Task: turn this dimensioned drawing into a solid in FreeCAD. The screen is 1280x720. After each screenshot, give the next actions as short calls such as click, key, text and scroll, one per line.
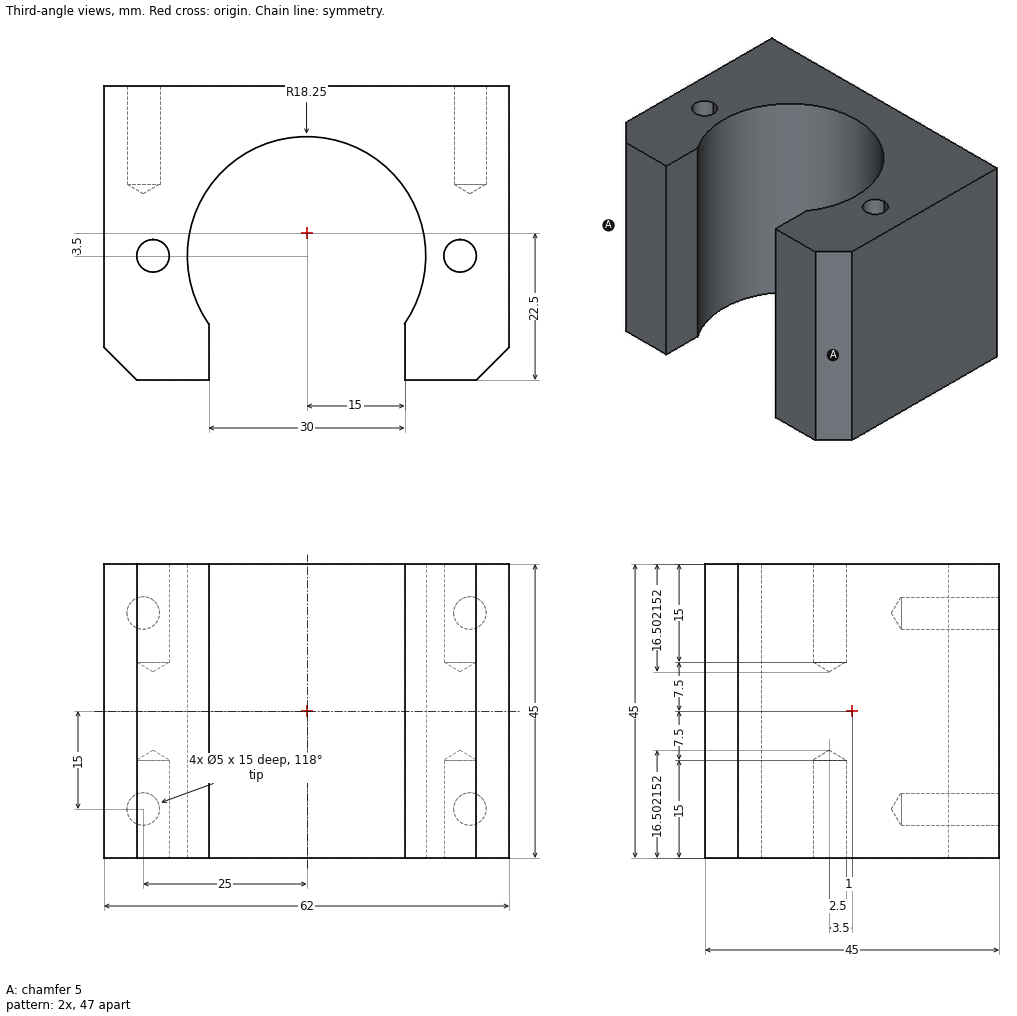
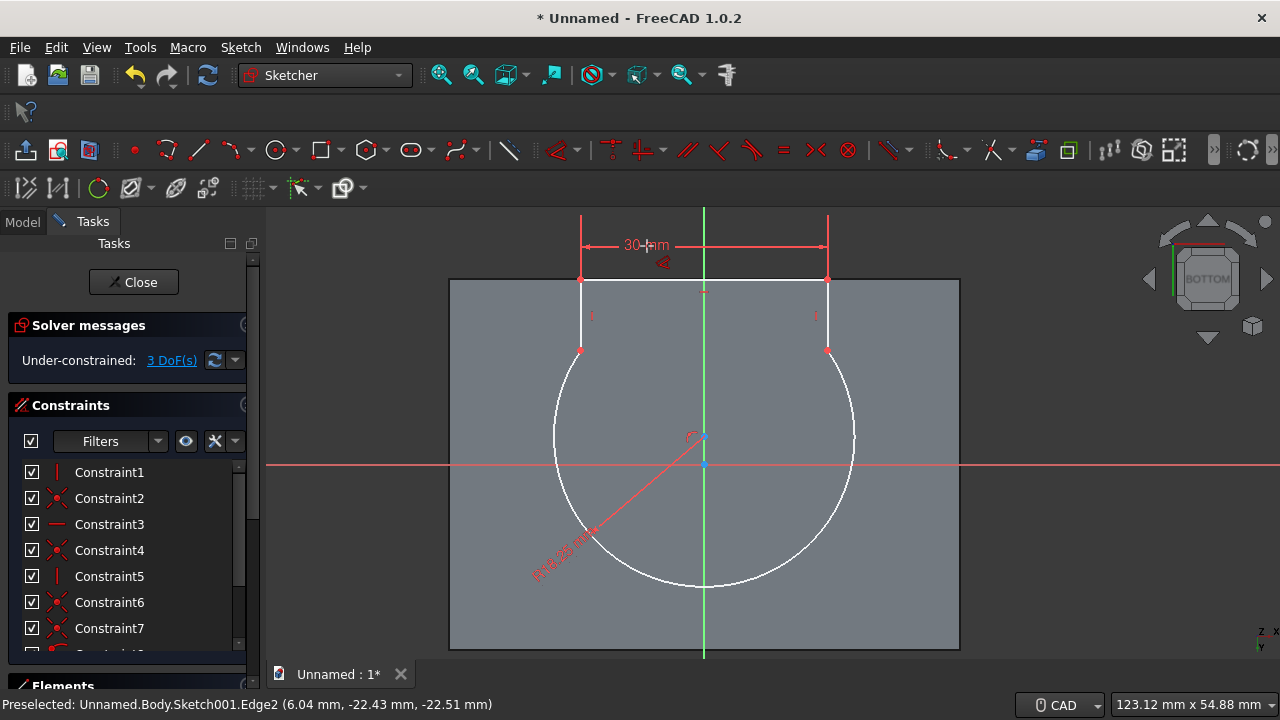
click(828, 351)
click(766, 317)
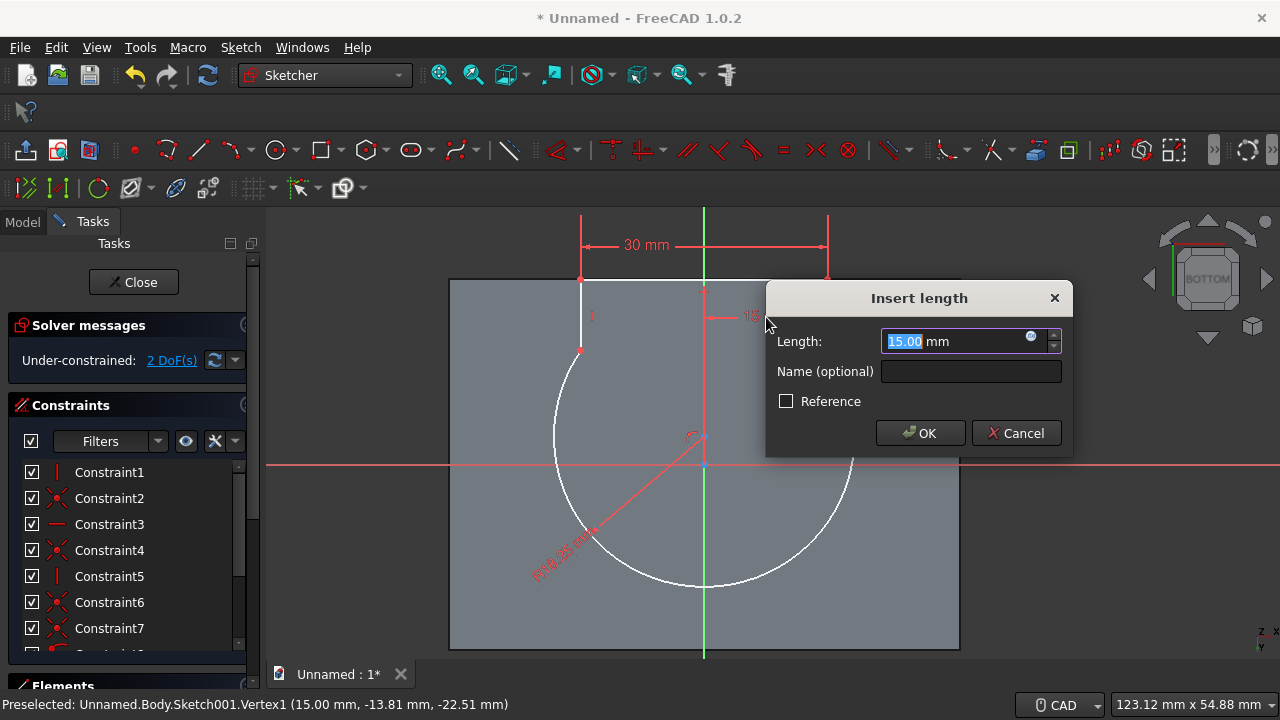
text(15)
key(Return)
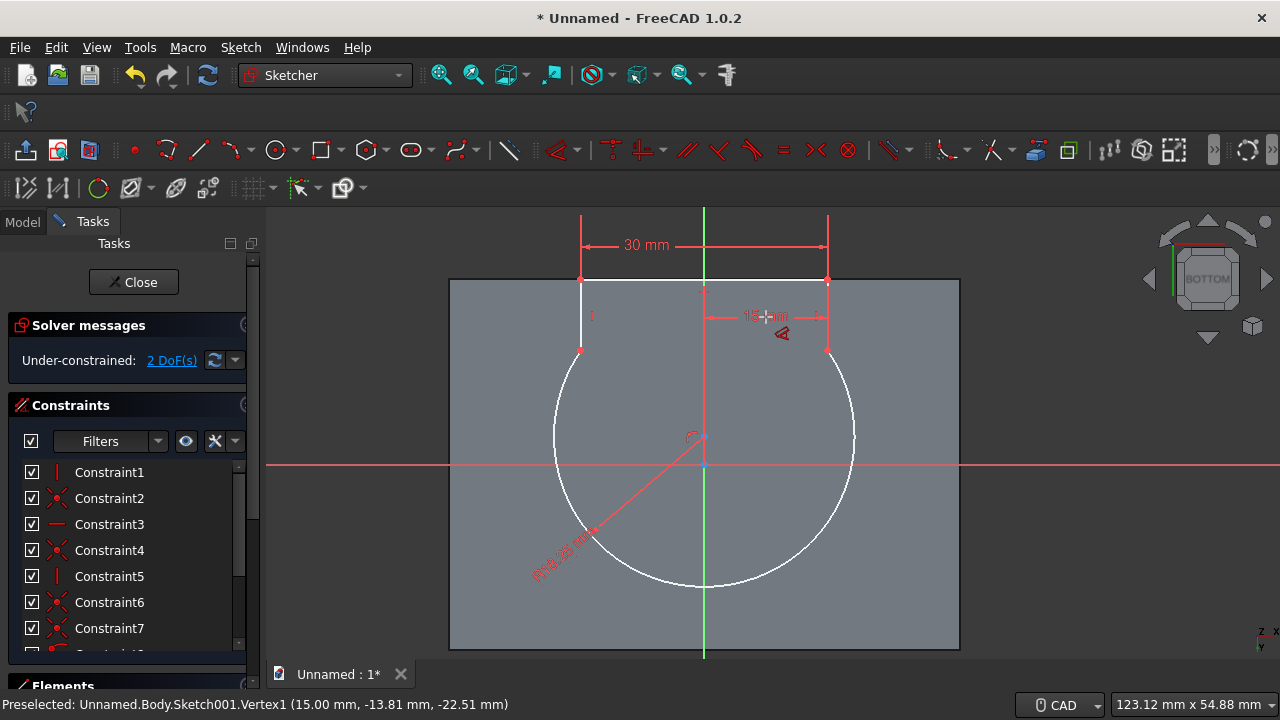
scroll(704, 437, up, 2)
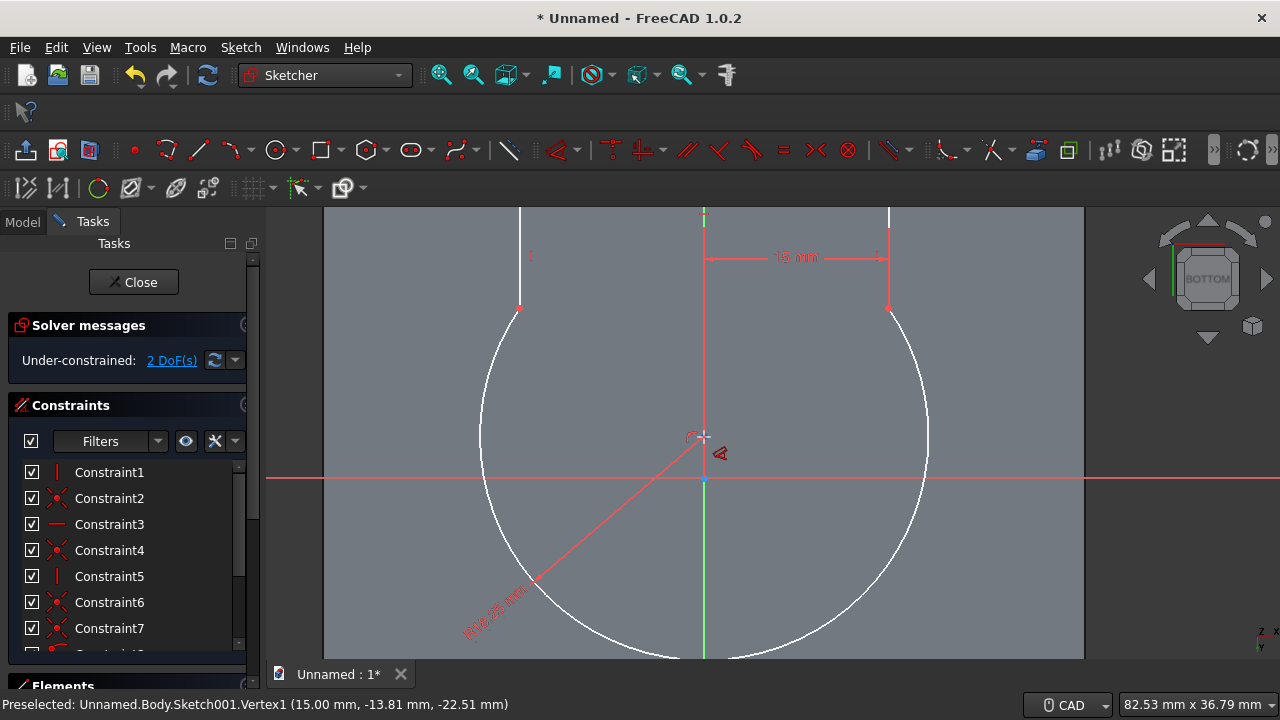
click(704, 436)
click(738, 457)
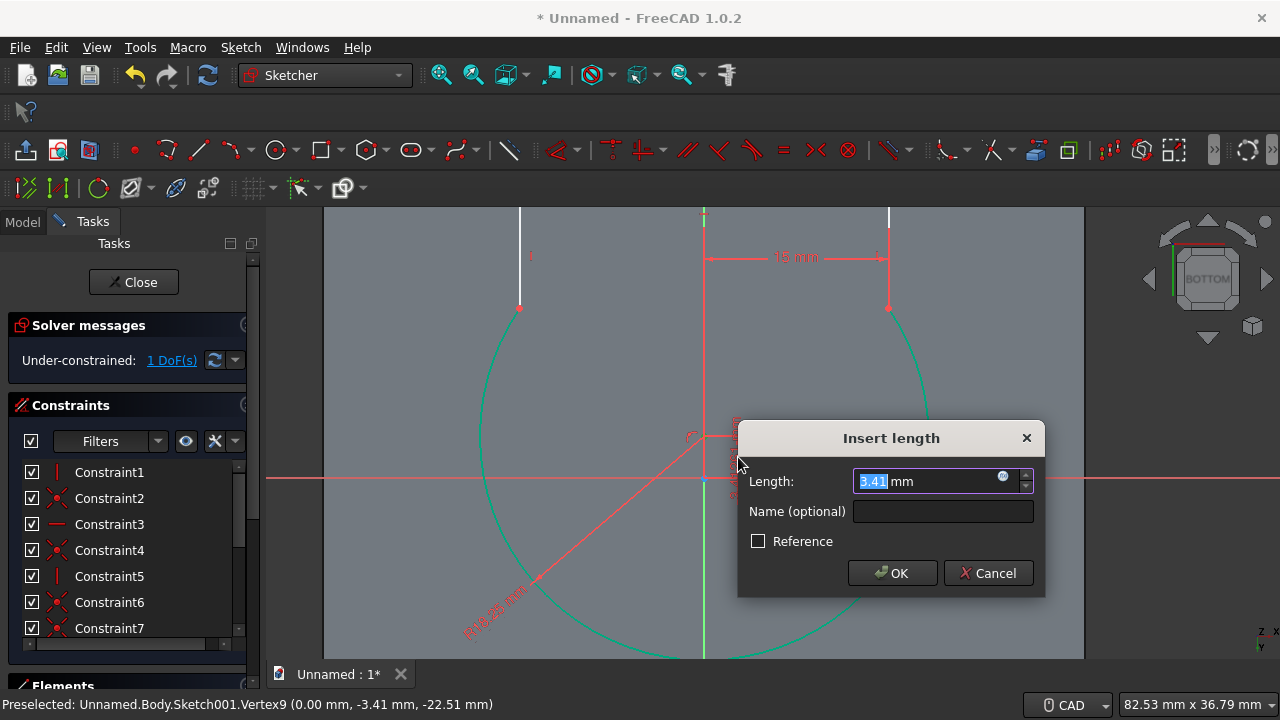
text(3.5)
key(Return)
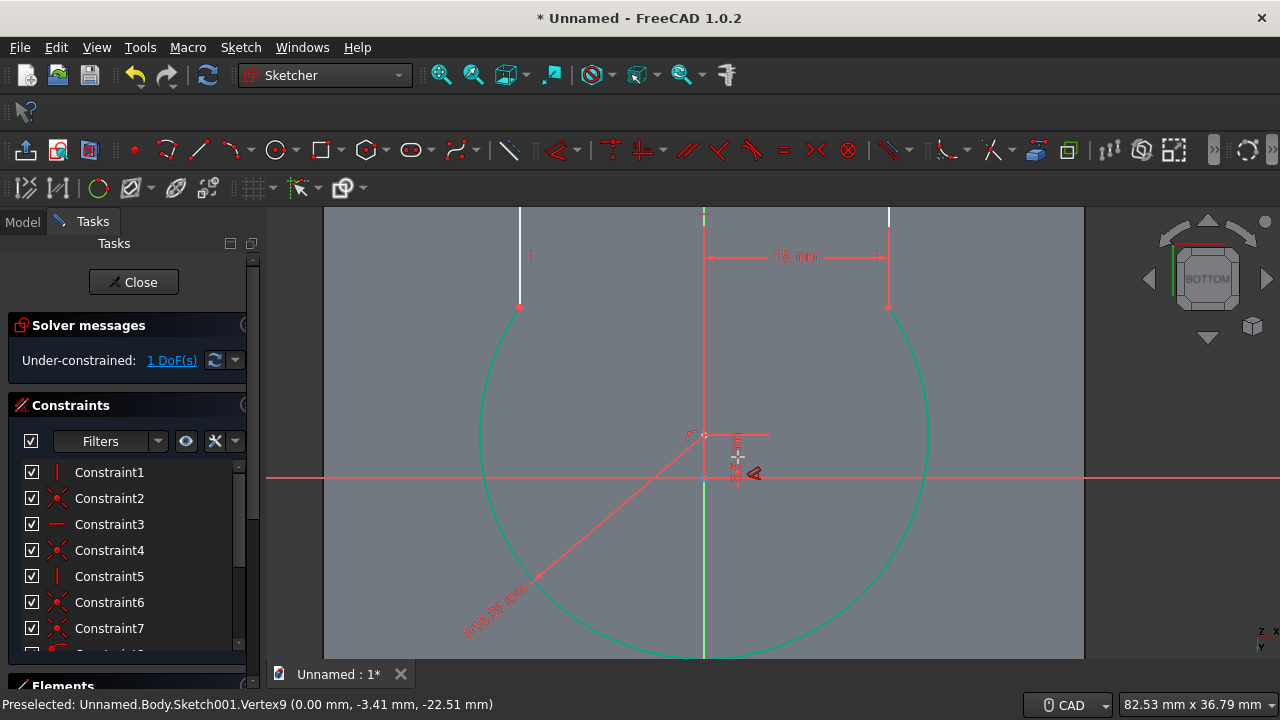
scroll(705, 438, down, 2)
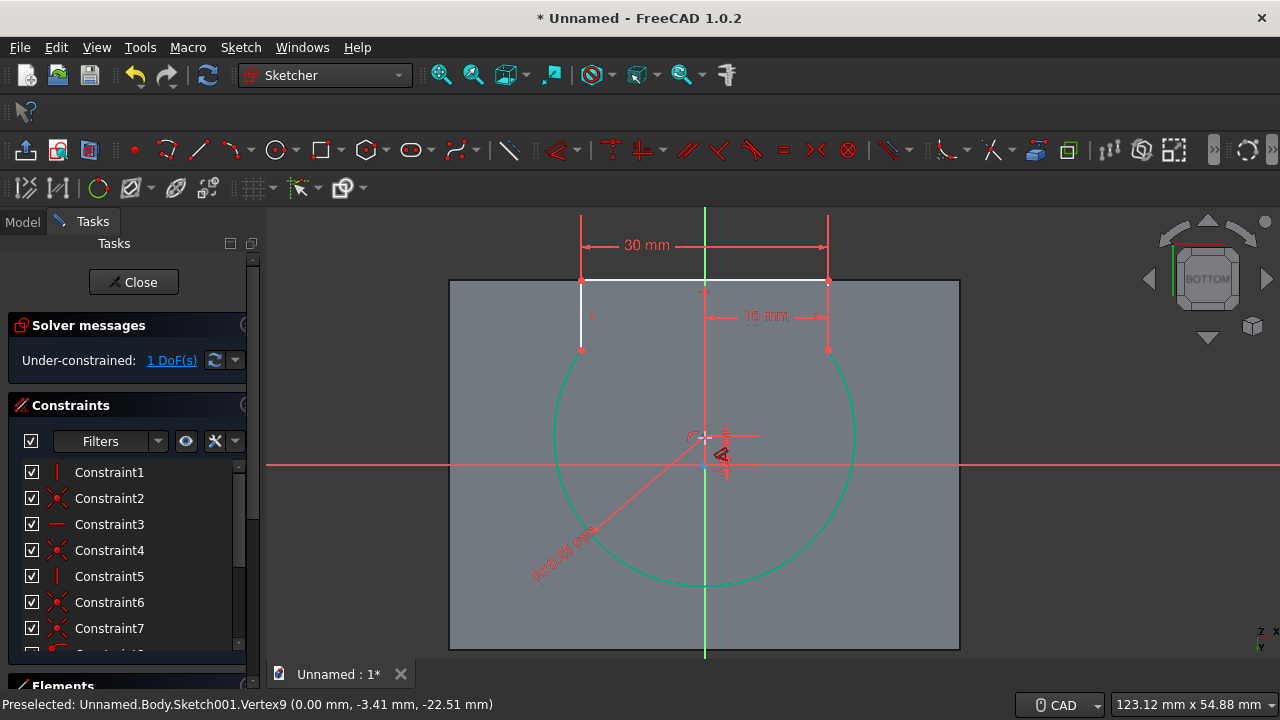
click(828, 280)
click(862, 373)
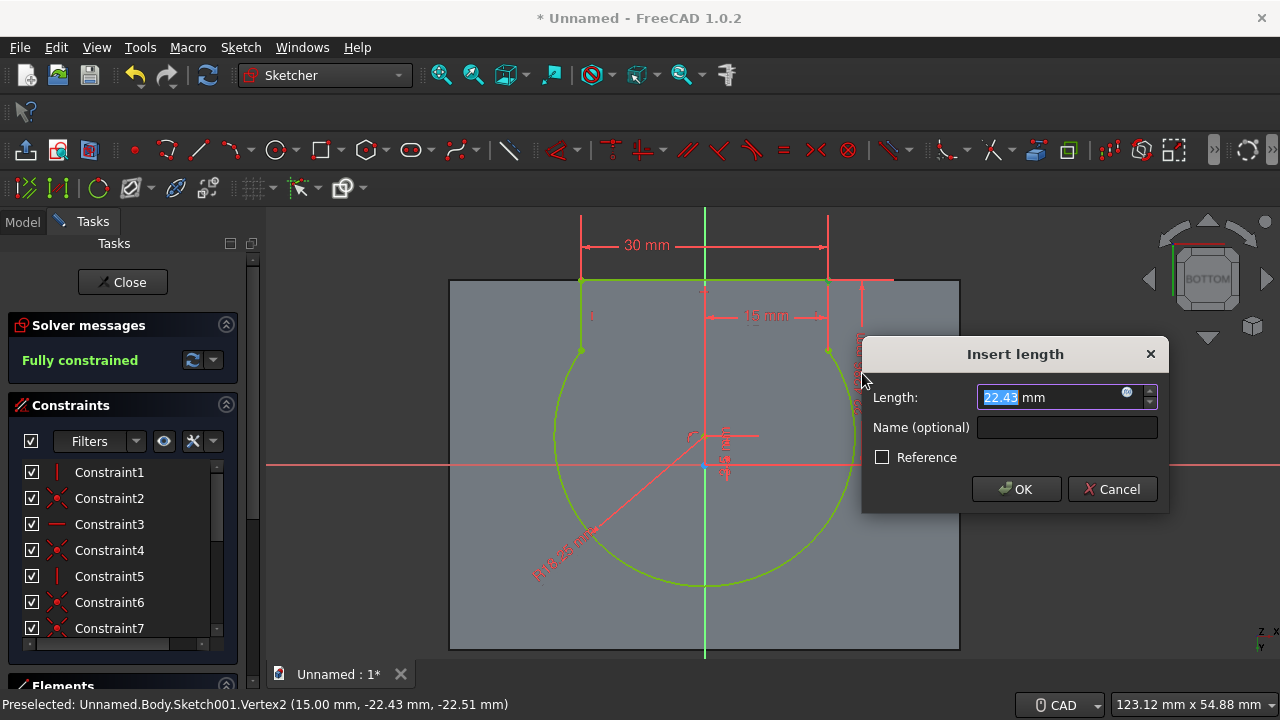
text(22.5)
key(Return)
key(Escape)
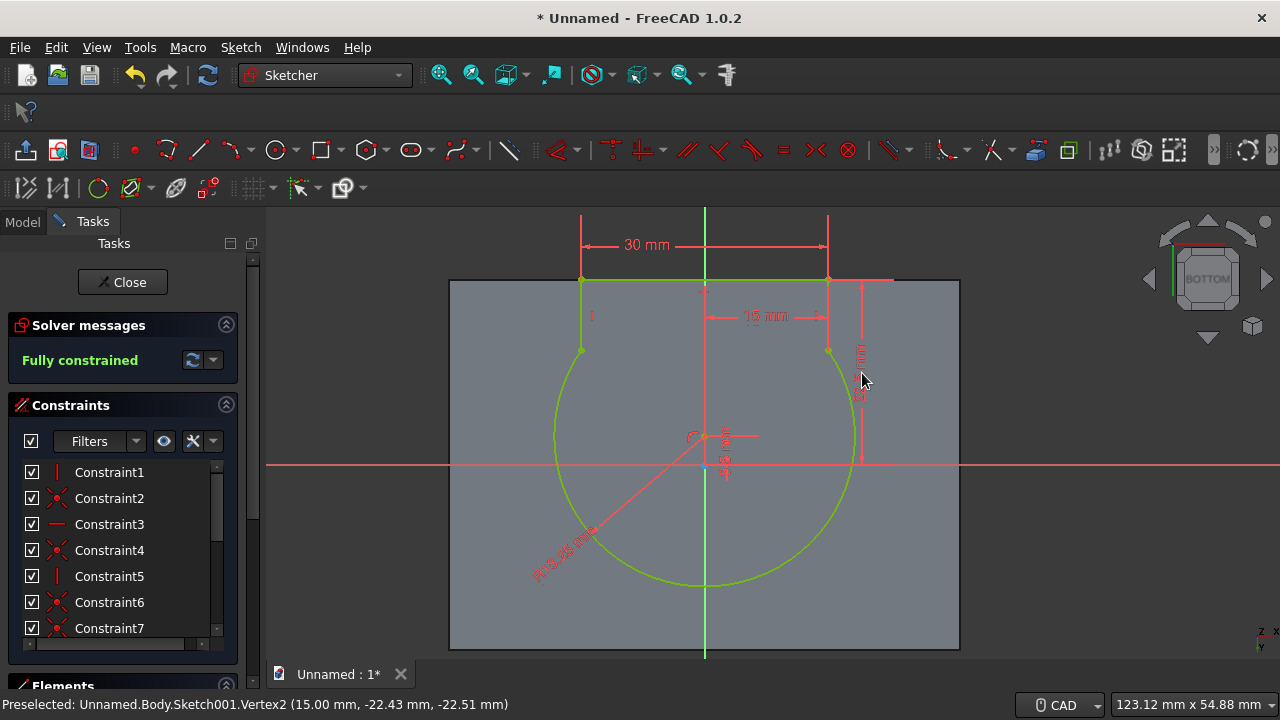
click(123, 282)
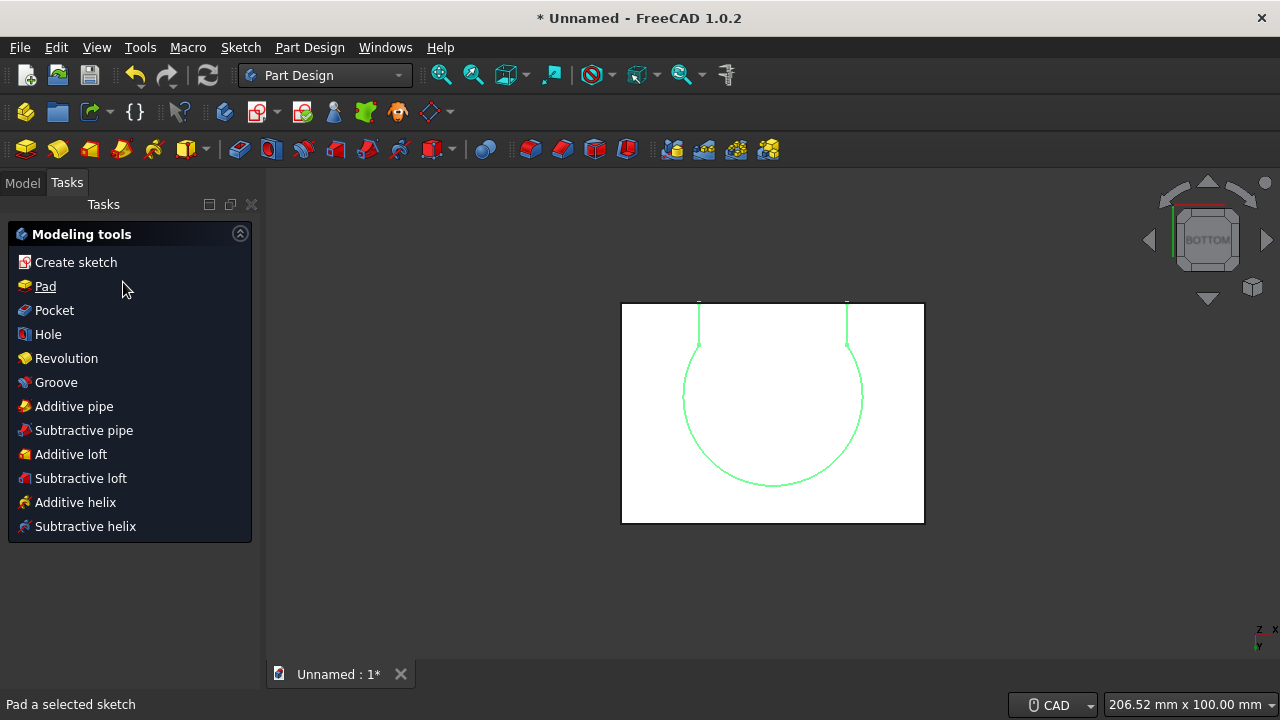
click(240, 150)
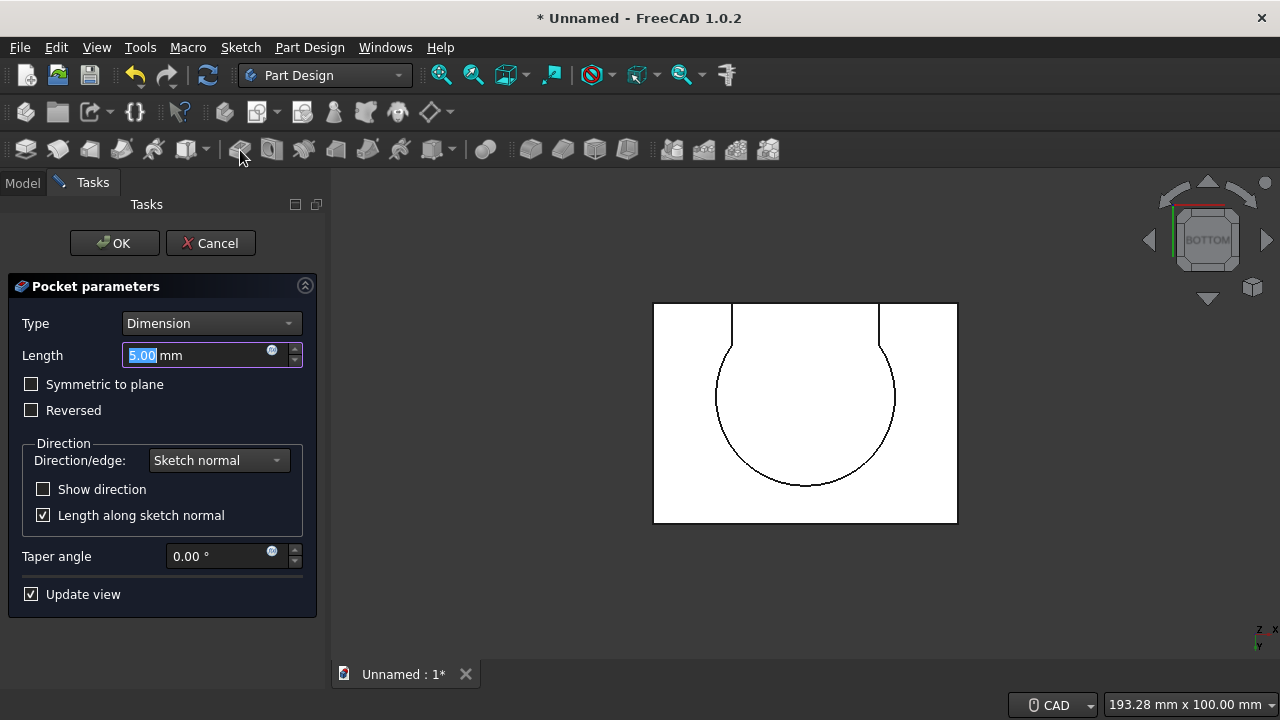
text(45)
key(Tab)